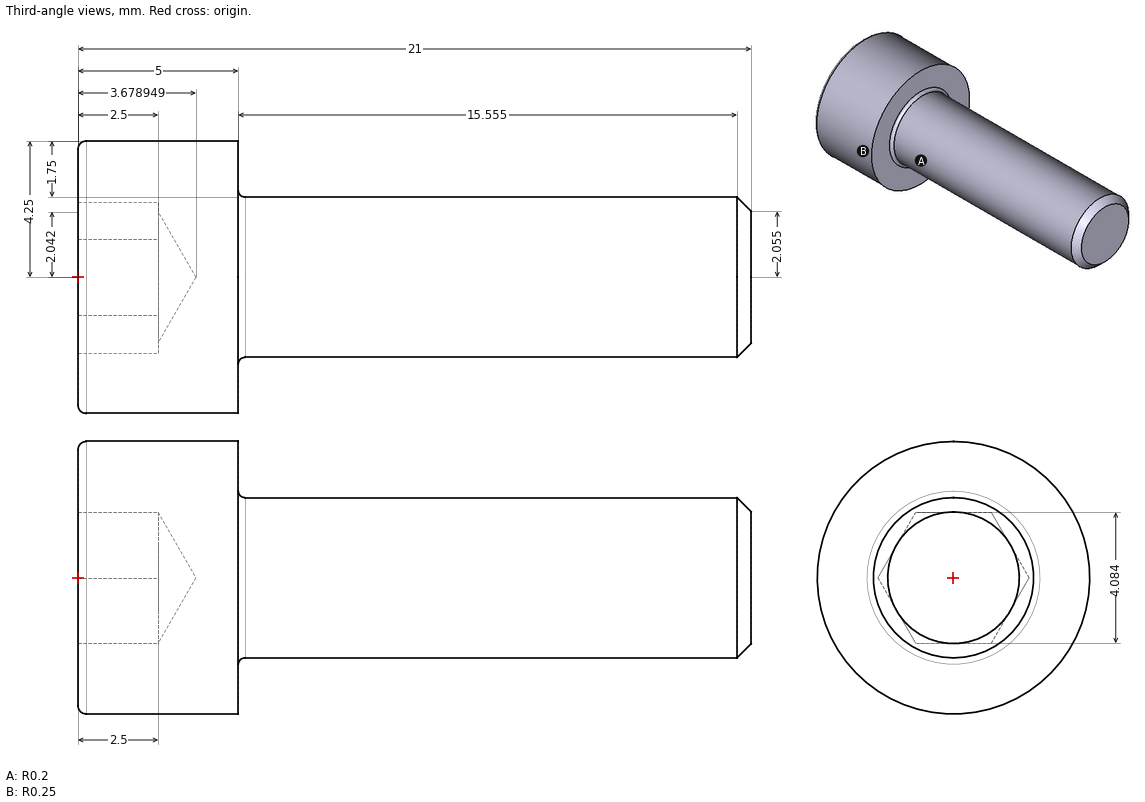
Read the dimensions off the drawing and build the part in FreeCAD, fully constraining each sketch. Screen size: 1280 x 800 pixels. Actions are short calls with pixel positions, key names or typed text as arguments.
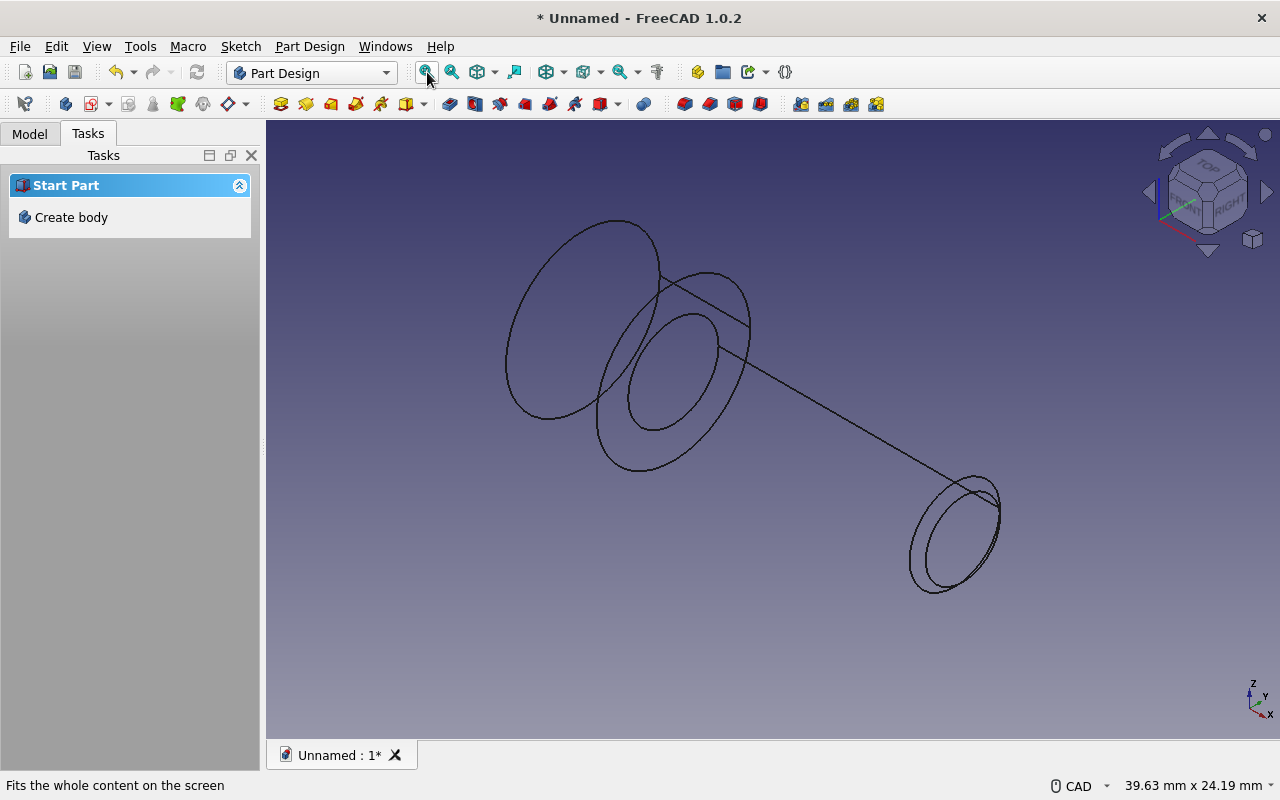
click(628, 397)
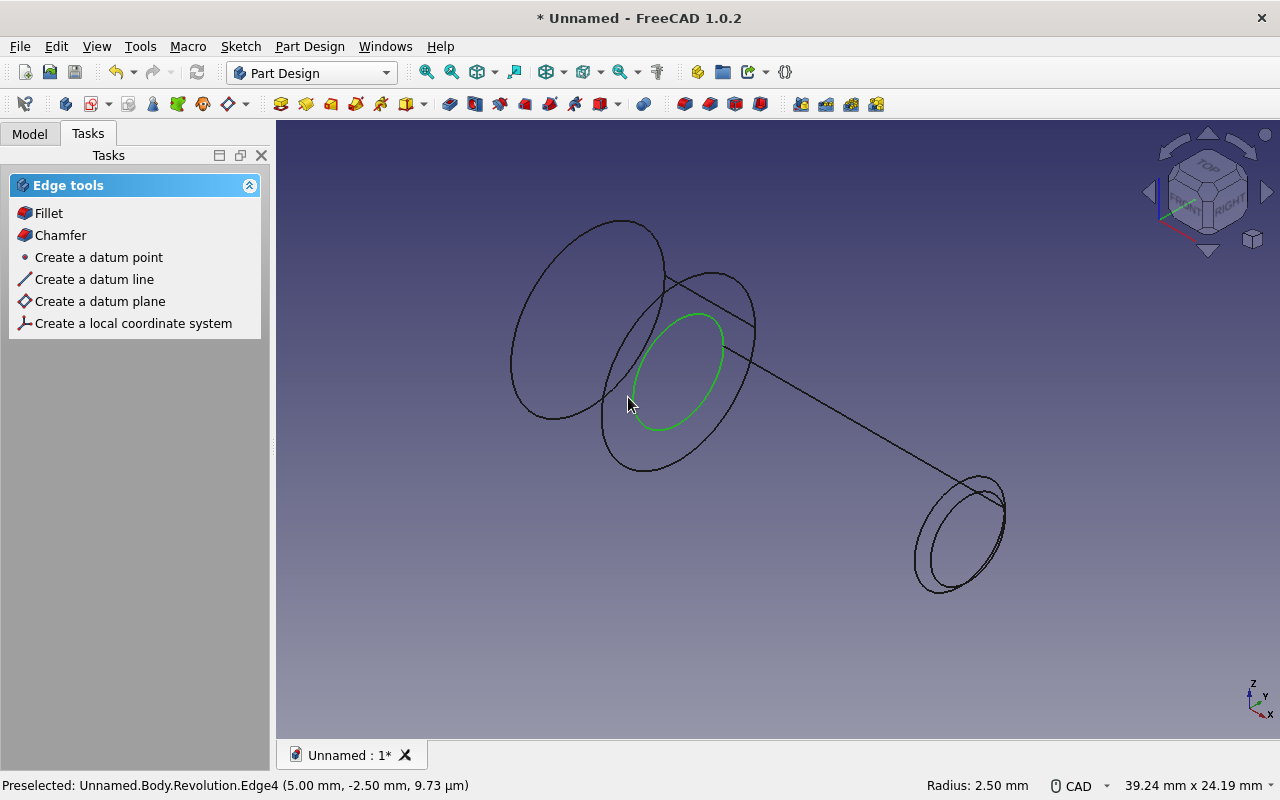
key(v)
key(1)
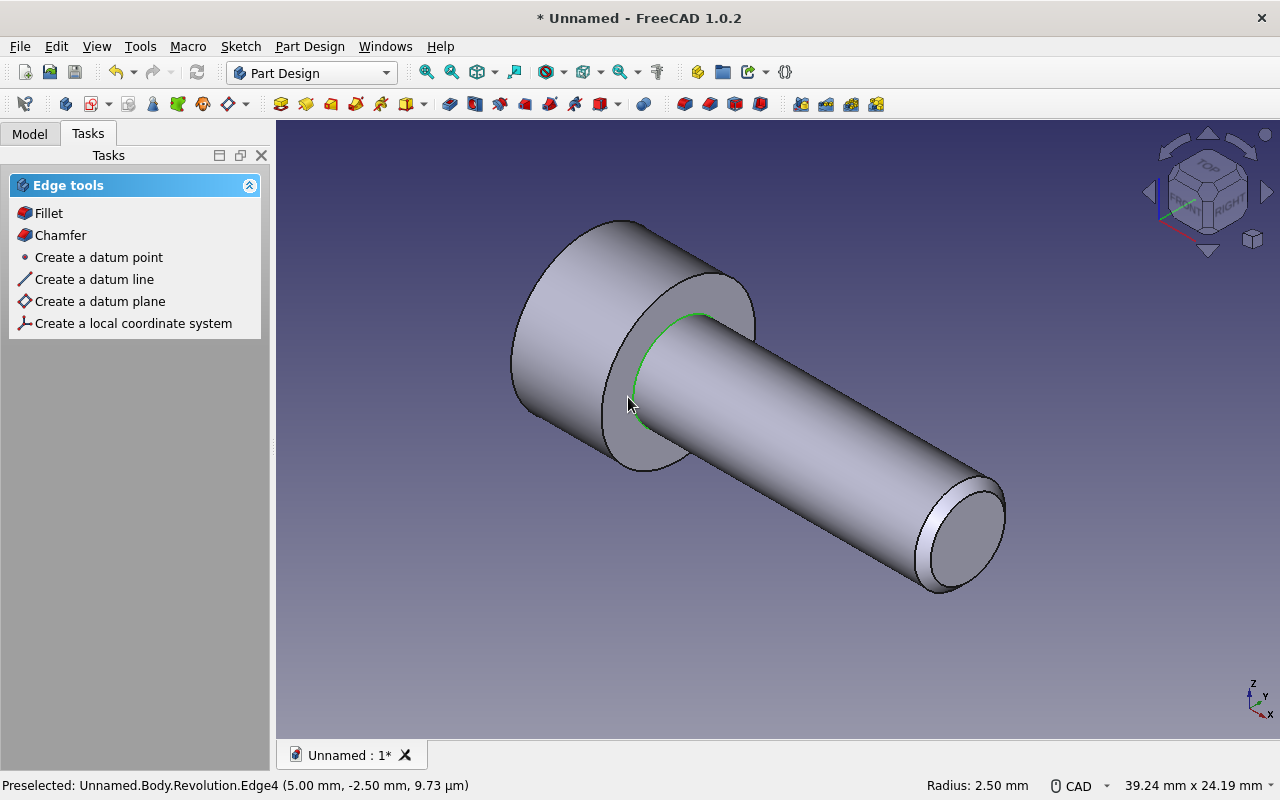
click(685, 104)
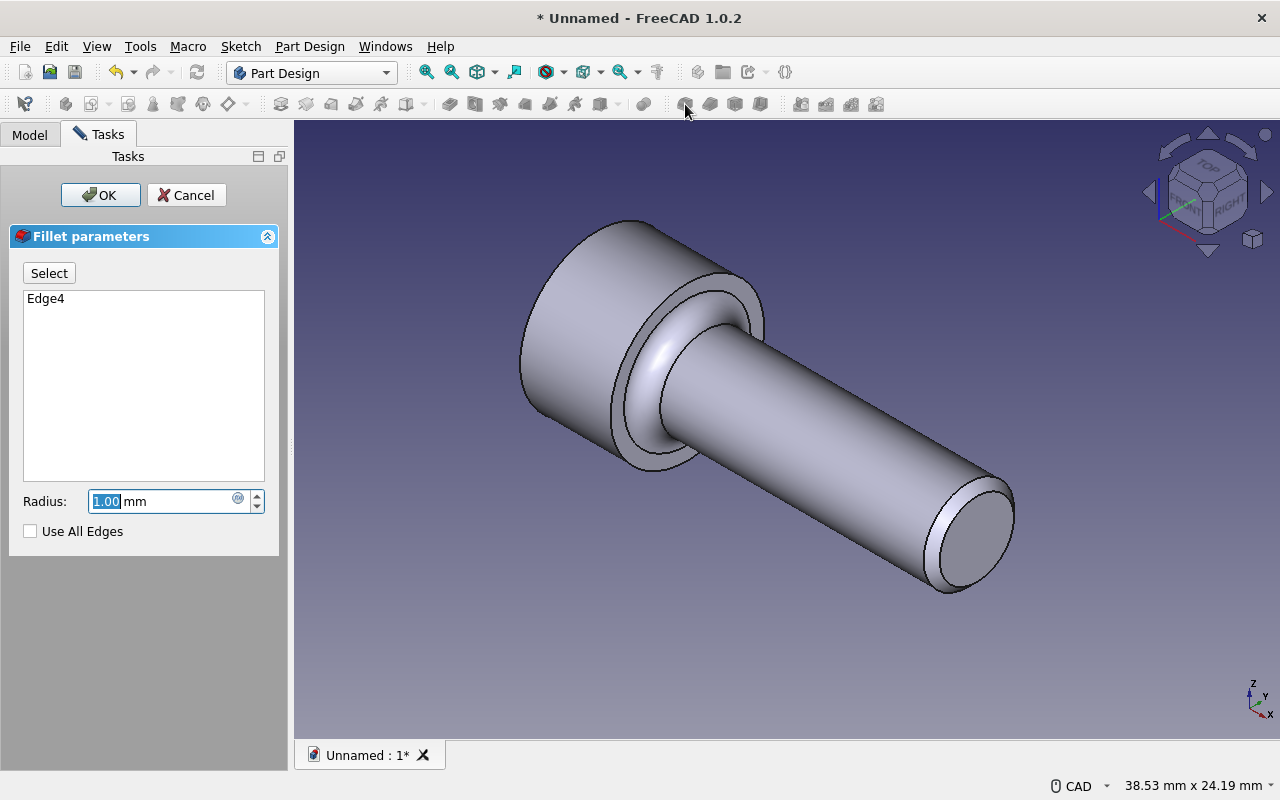
text(0.2)
key(Tab)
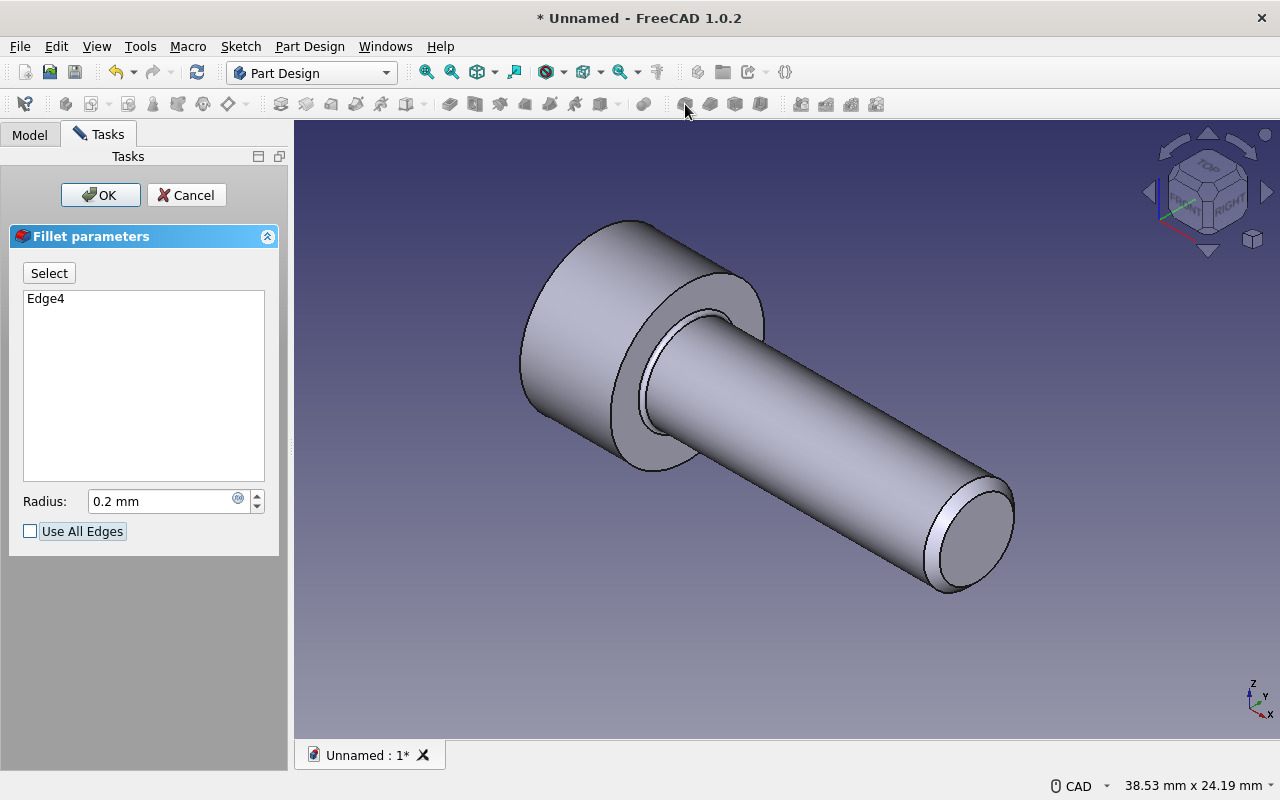
click(101, 195)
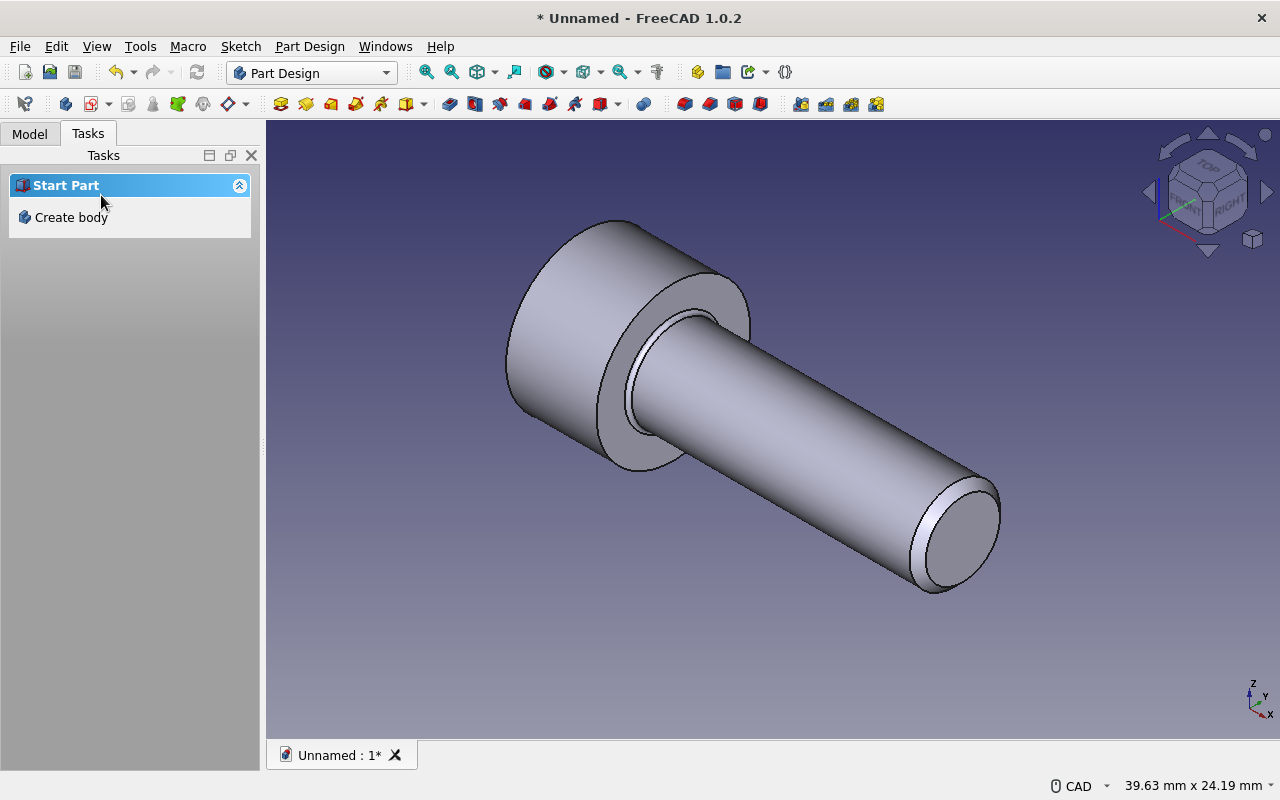
key(2)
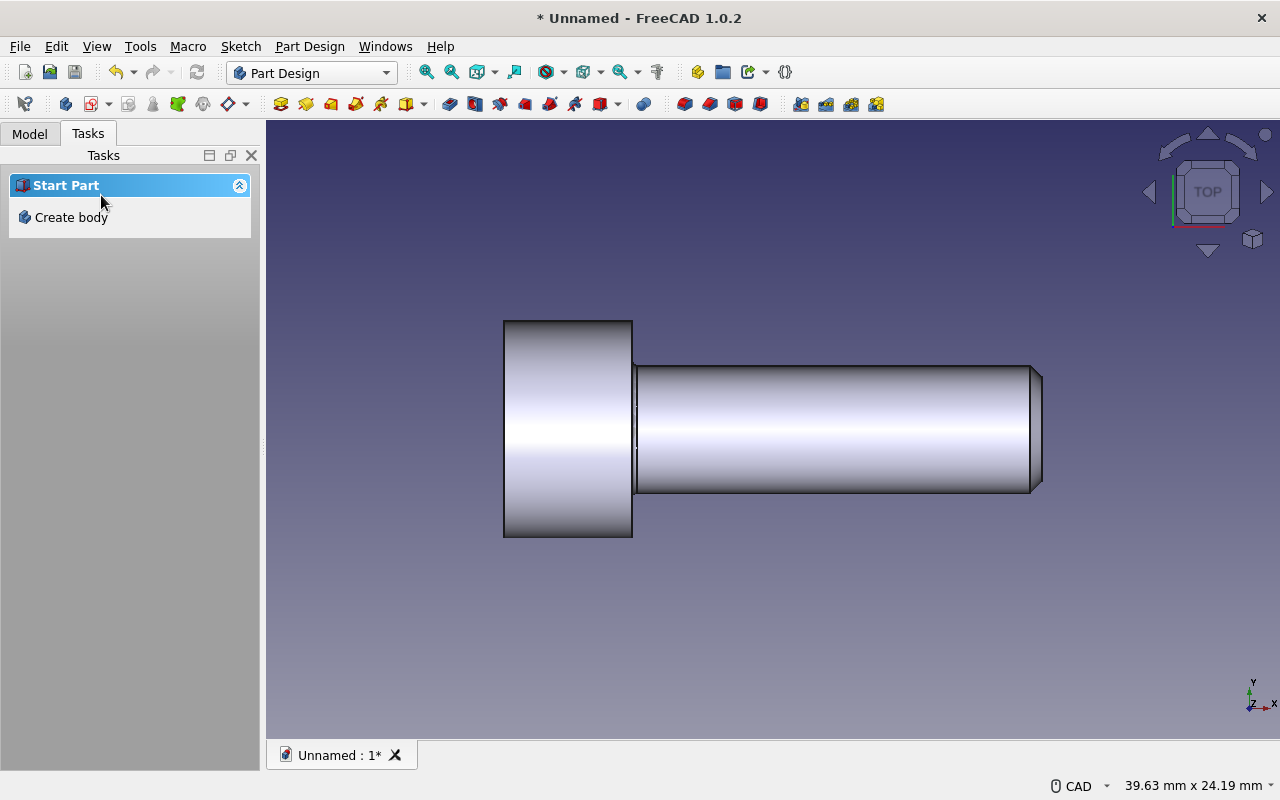
click(504, 517)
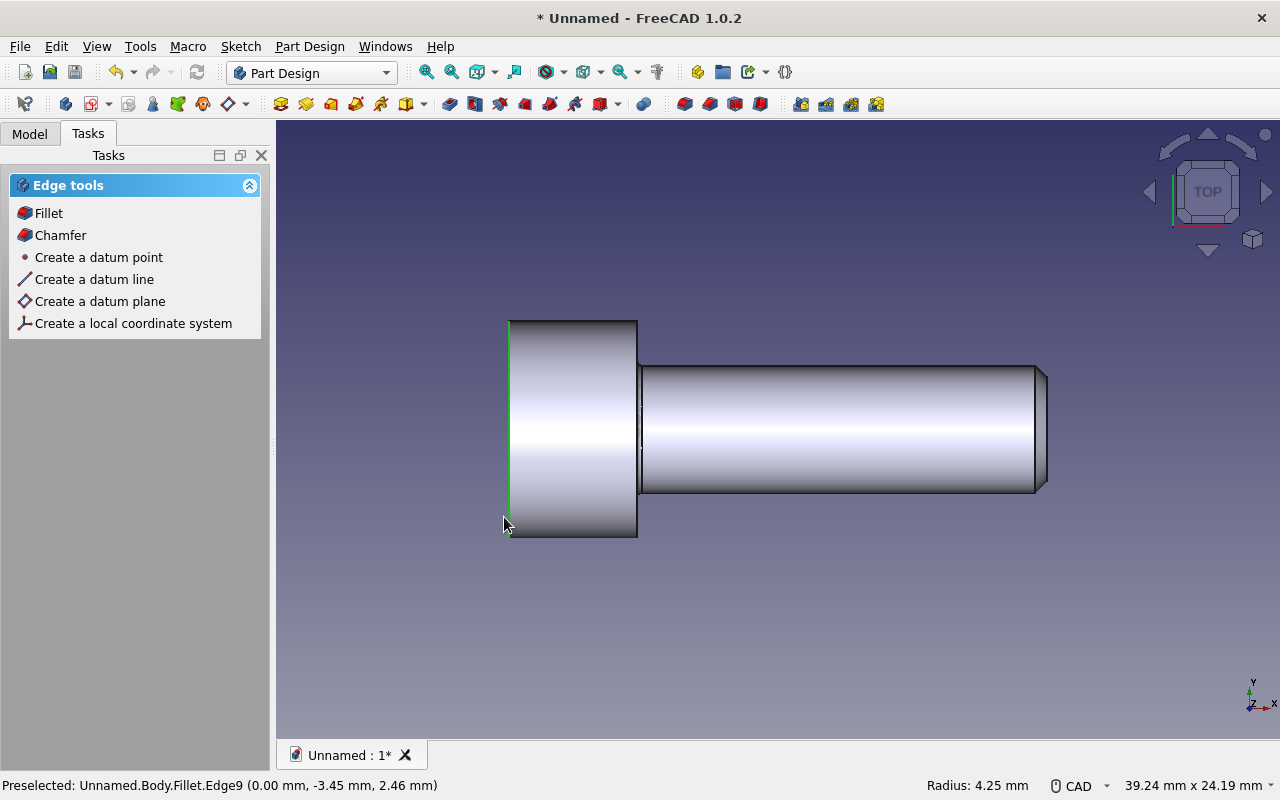
click(685, 104)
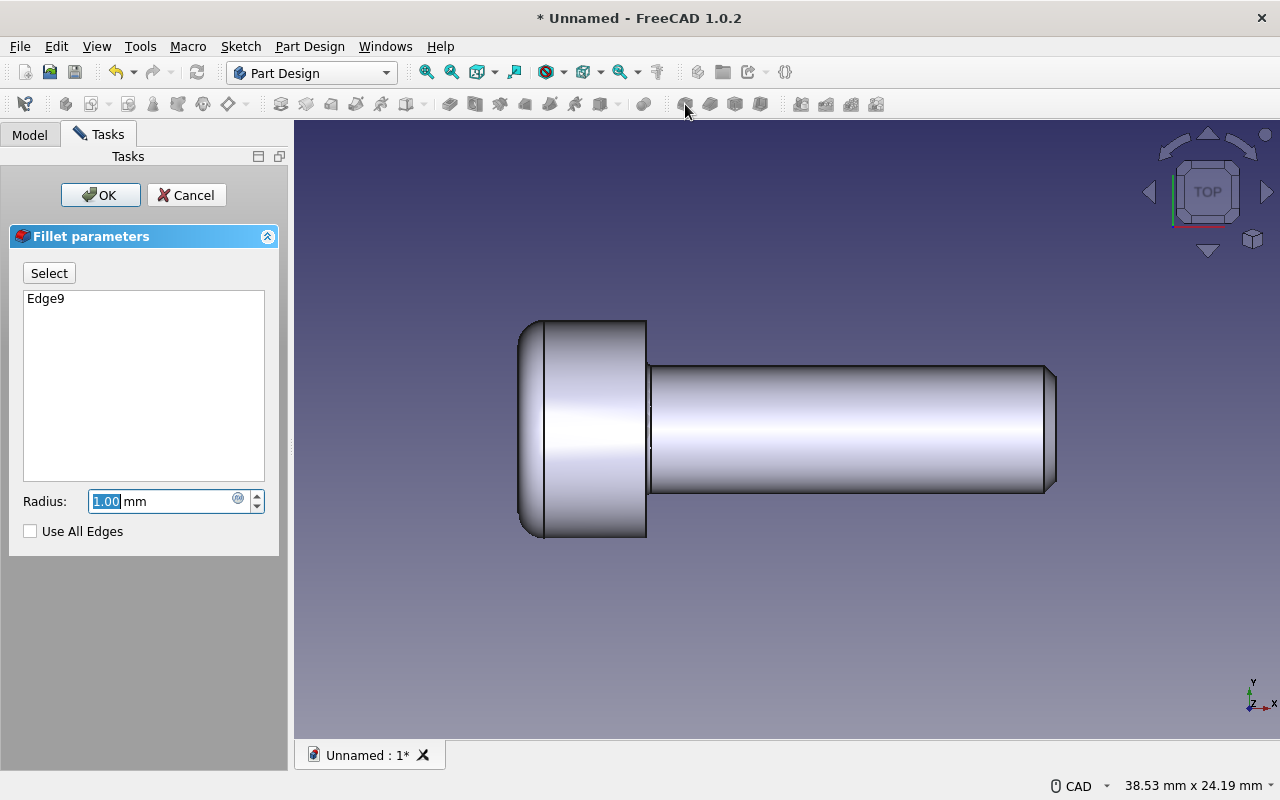
text(0.25)
key(Tab)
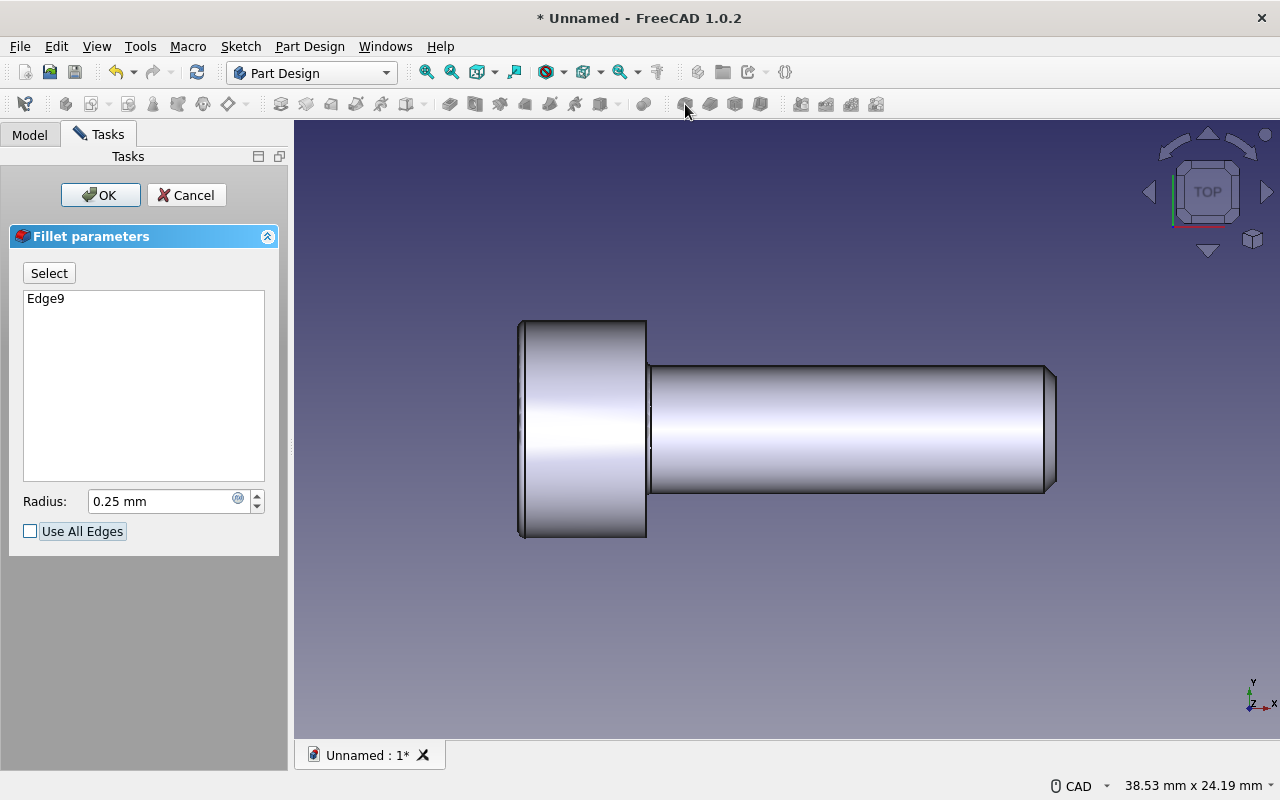
click(101, 195)